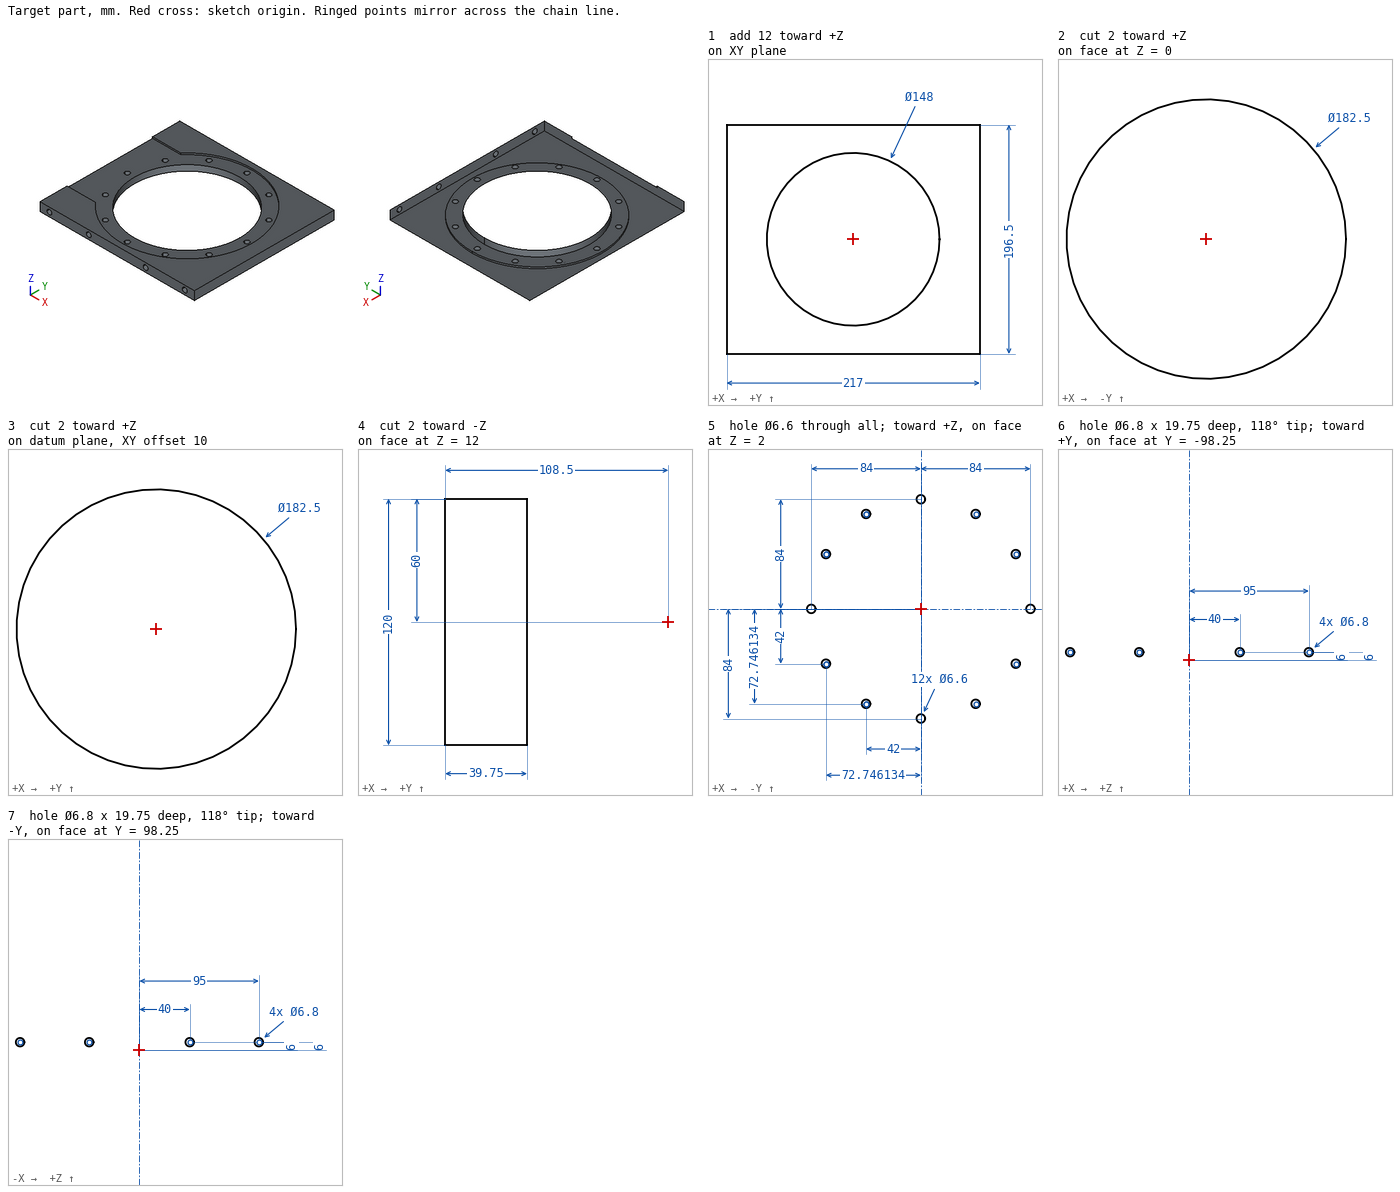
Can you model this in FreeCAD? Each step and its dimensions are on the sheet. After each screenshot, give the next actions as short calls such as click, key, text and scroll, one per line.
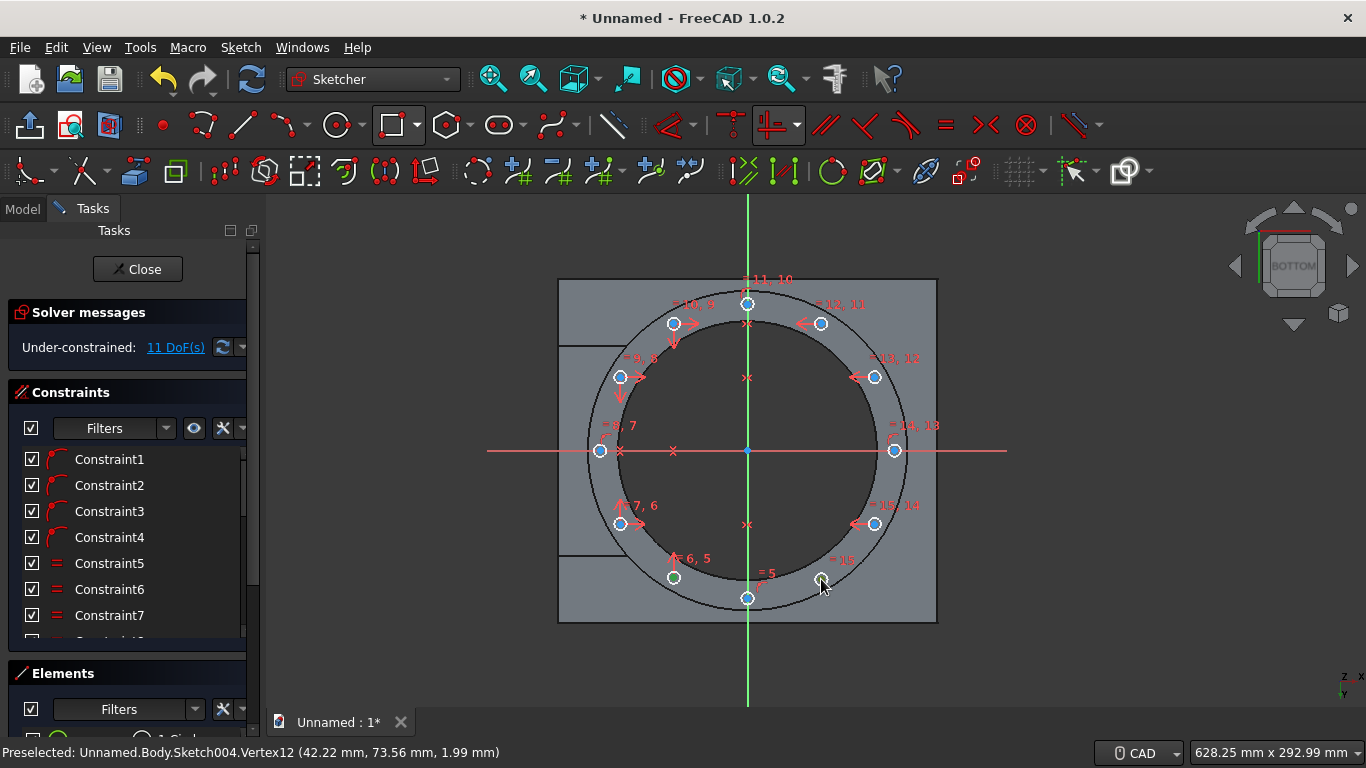
click(748, 646)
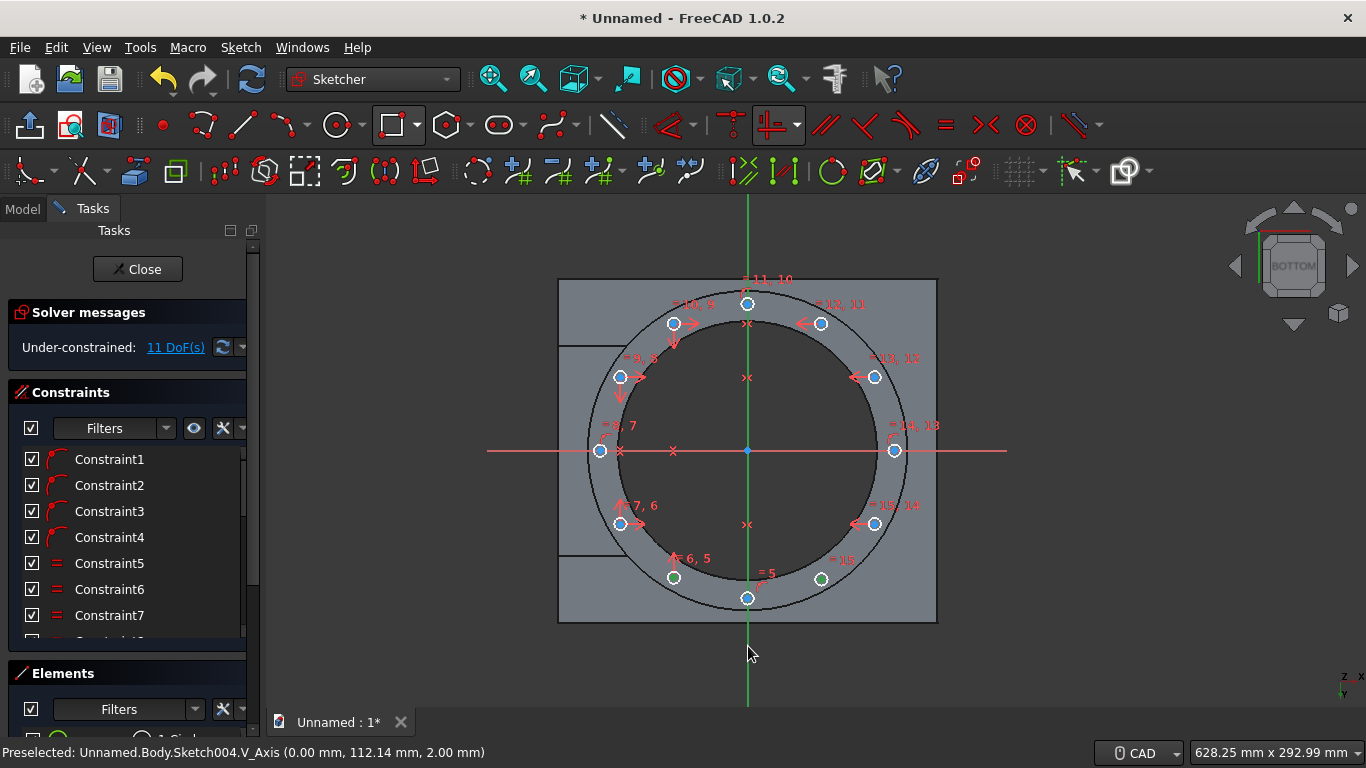
click(986, 126)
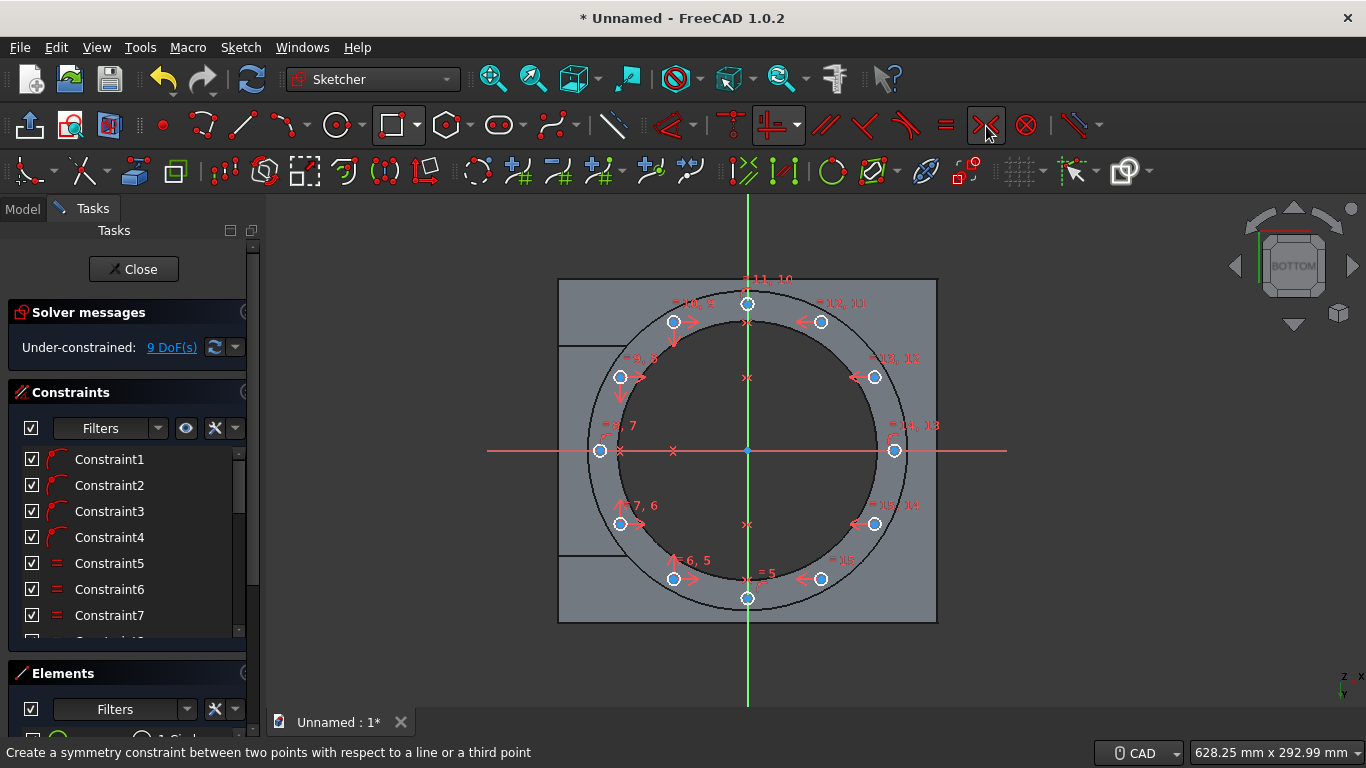
click(668, 126)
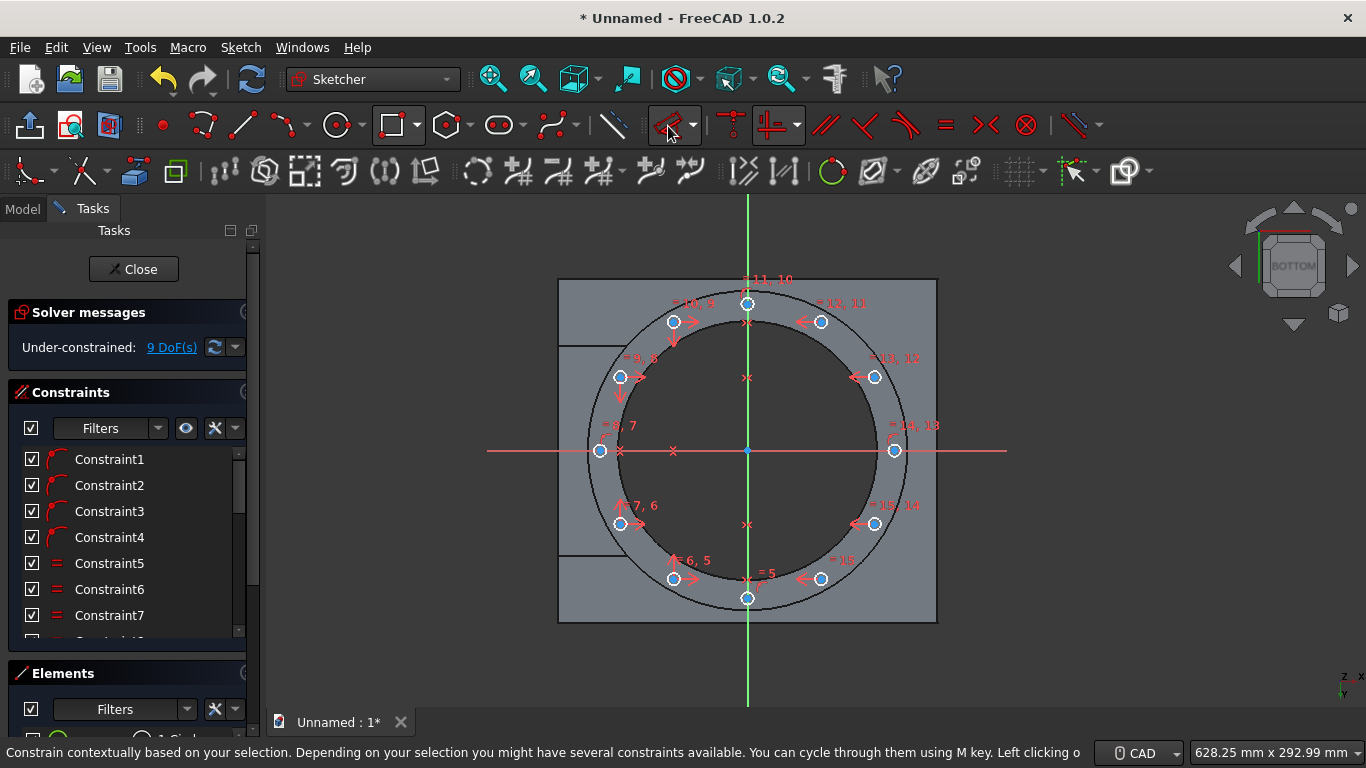
scroll(748, 592, up, 7)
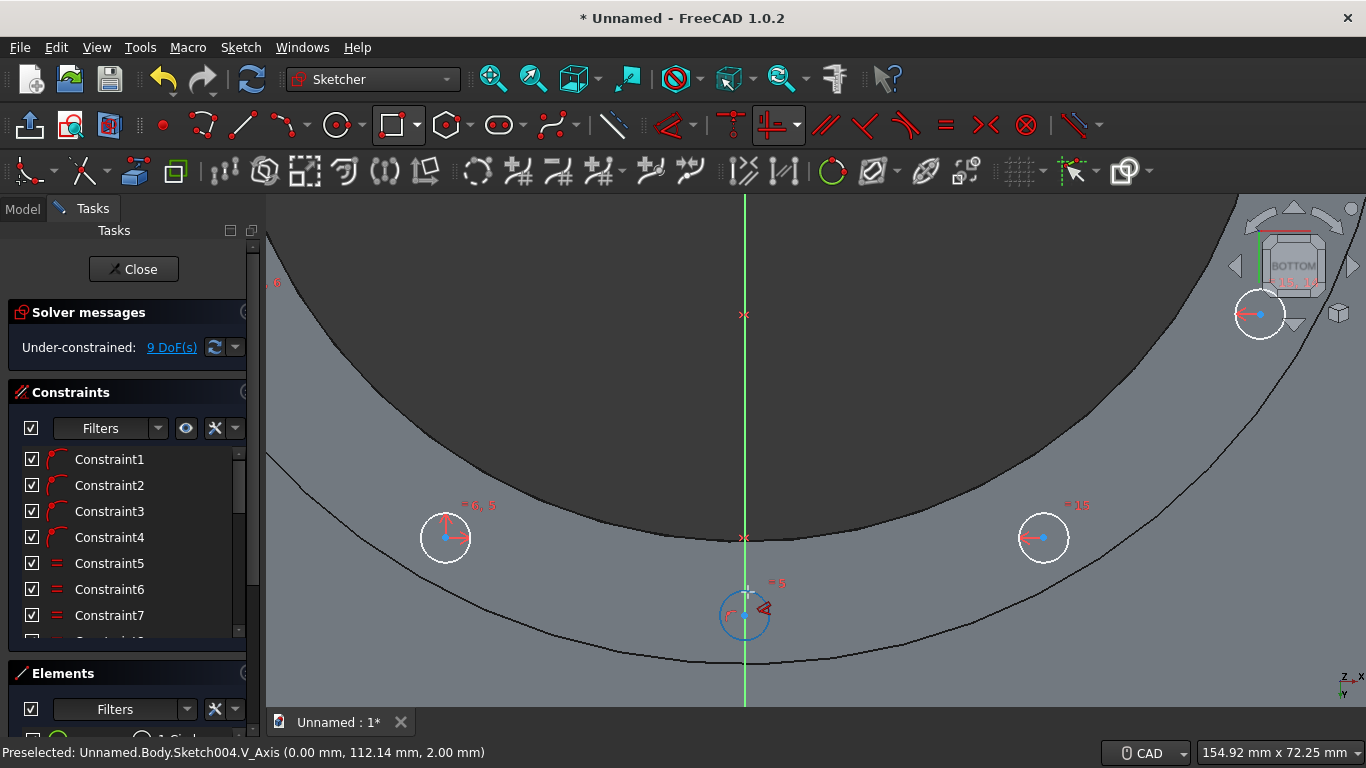
click(745, 591)
click(772, 566)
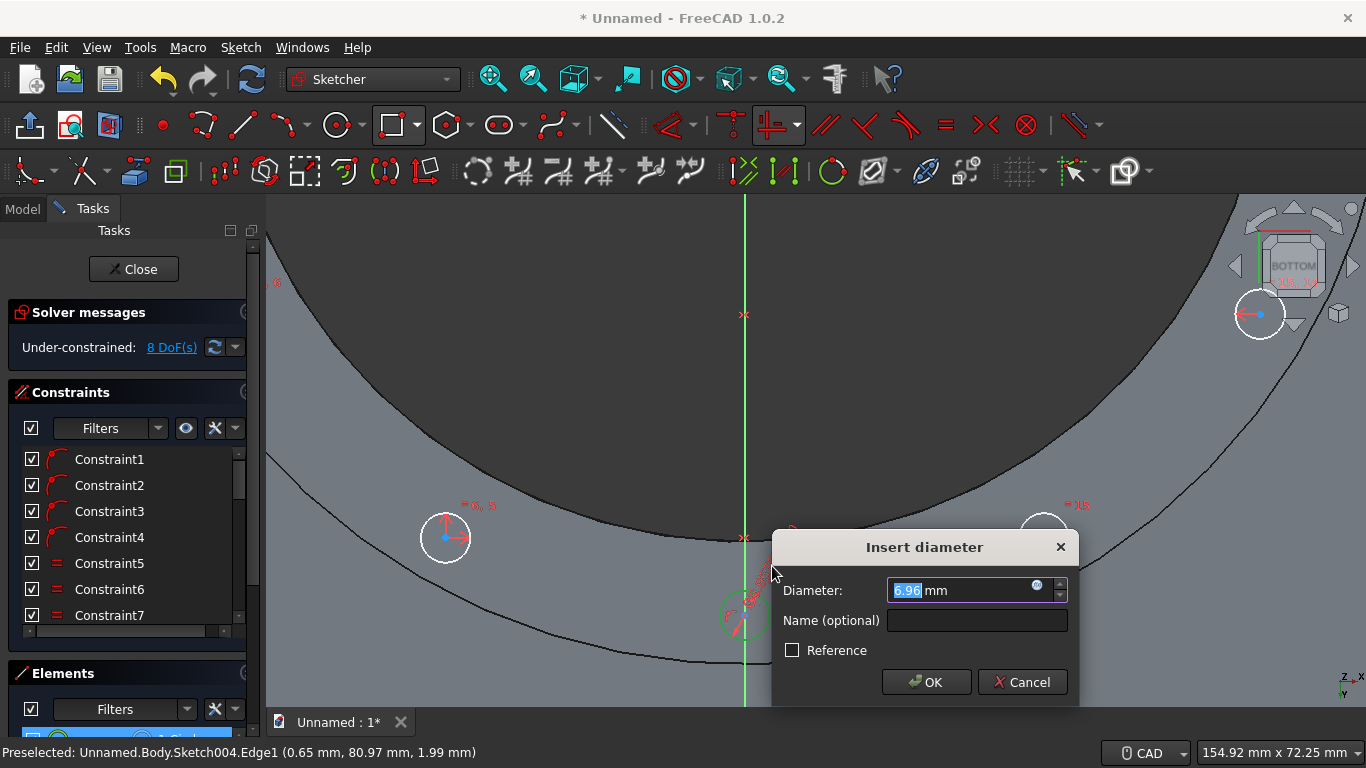
text(6.6)
key(Return)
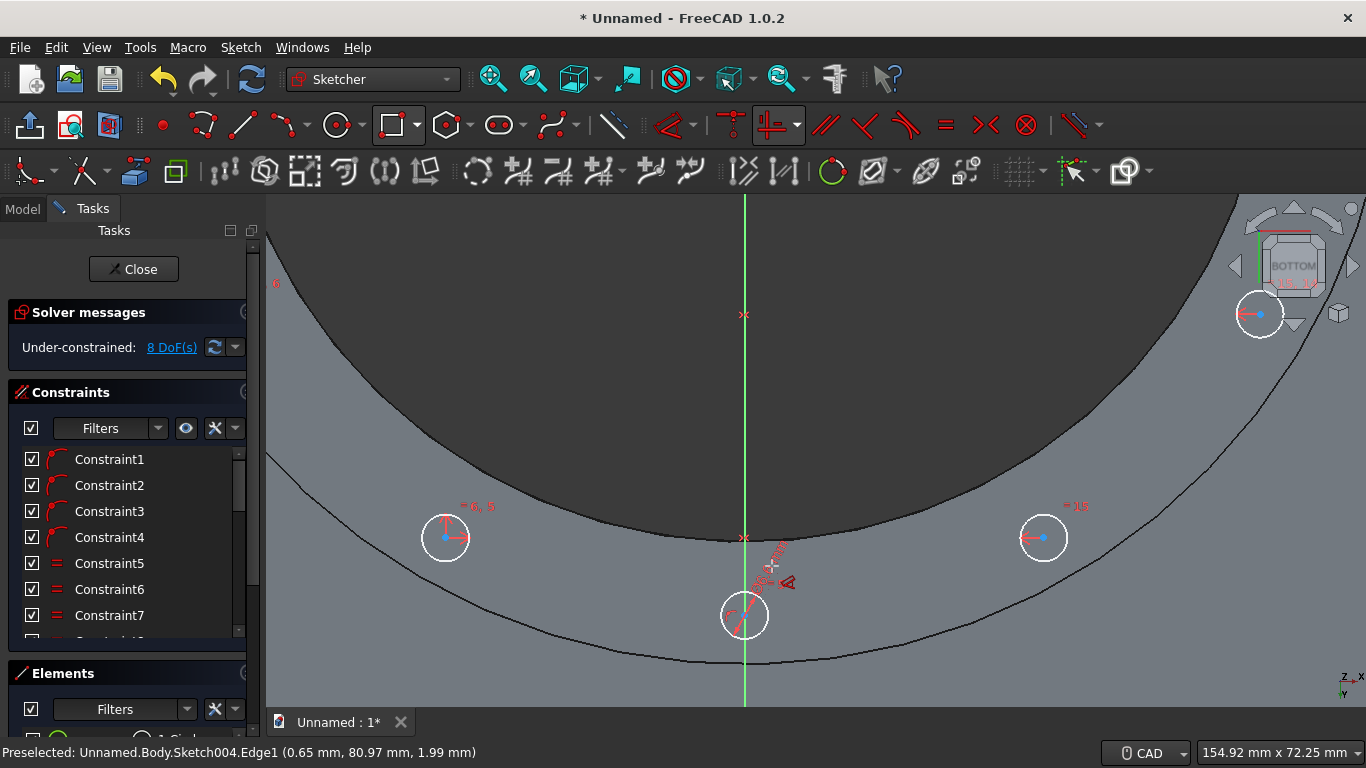
scroll(748, 593, down, 7)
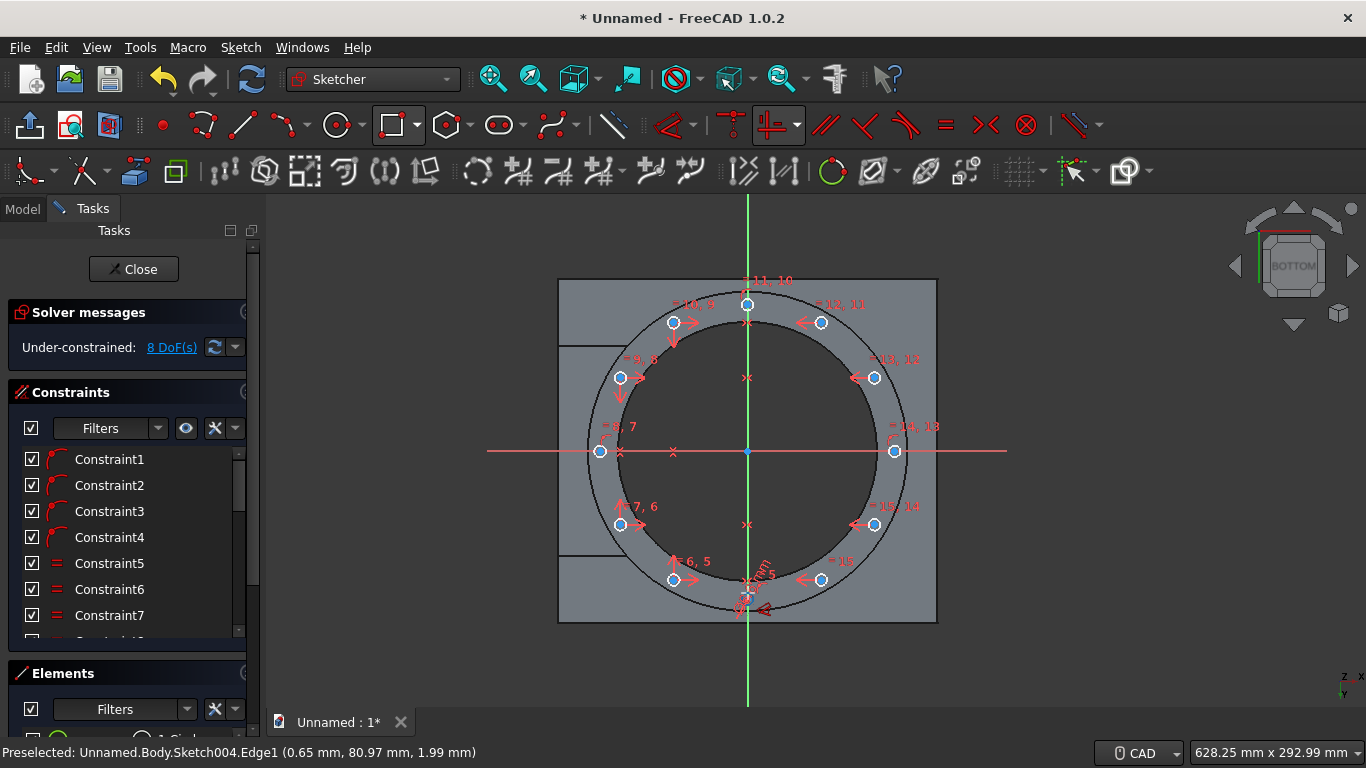
click(748, 599)
click(782, 525)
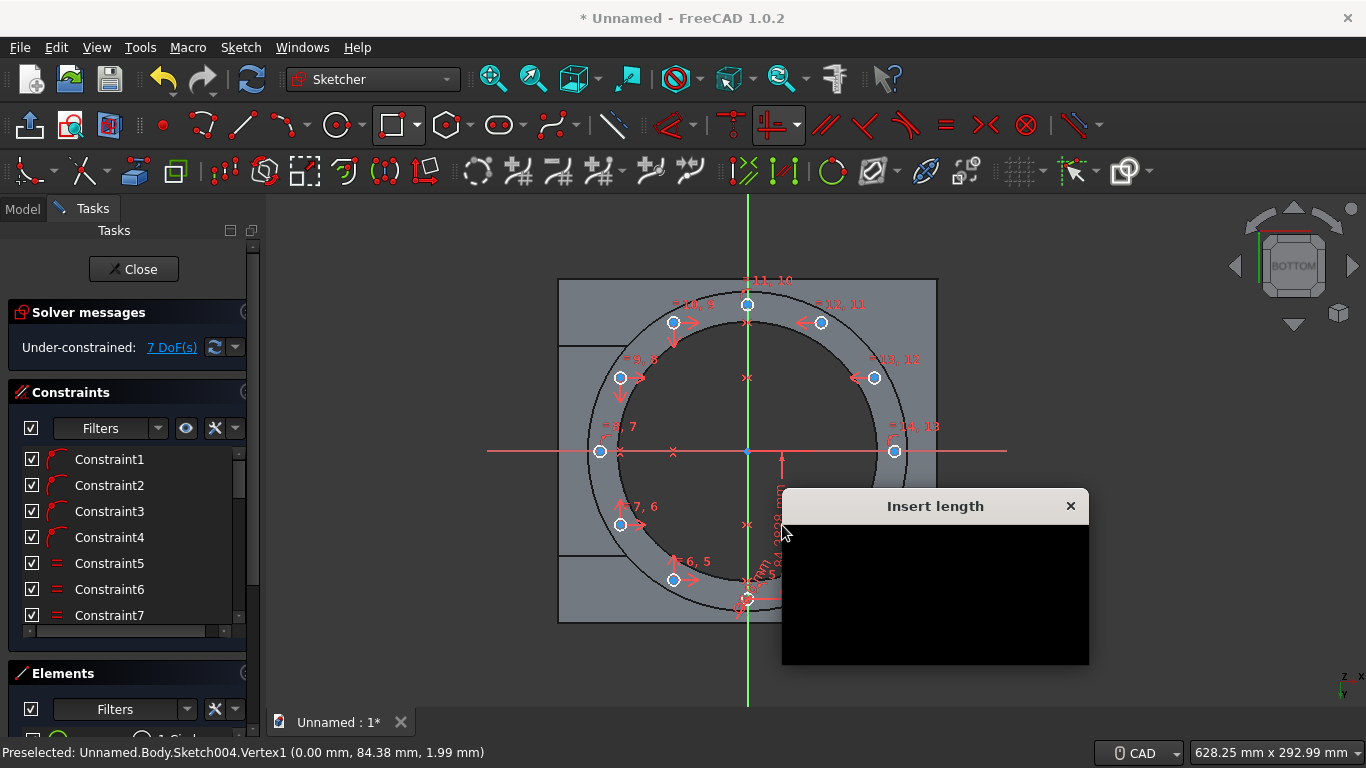
text(84)
key(Return)